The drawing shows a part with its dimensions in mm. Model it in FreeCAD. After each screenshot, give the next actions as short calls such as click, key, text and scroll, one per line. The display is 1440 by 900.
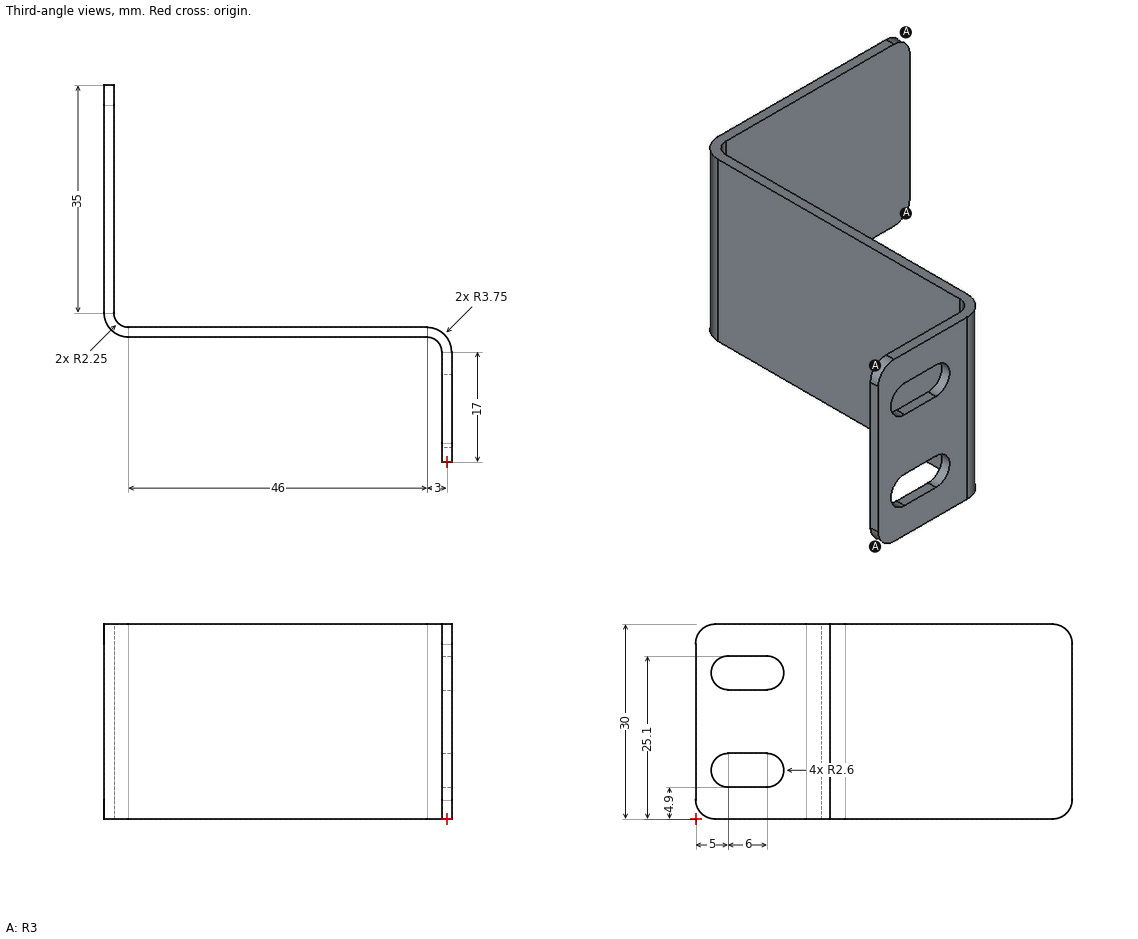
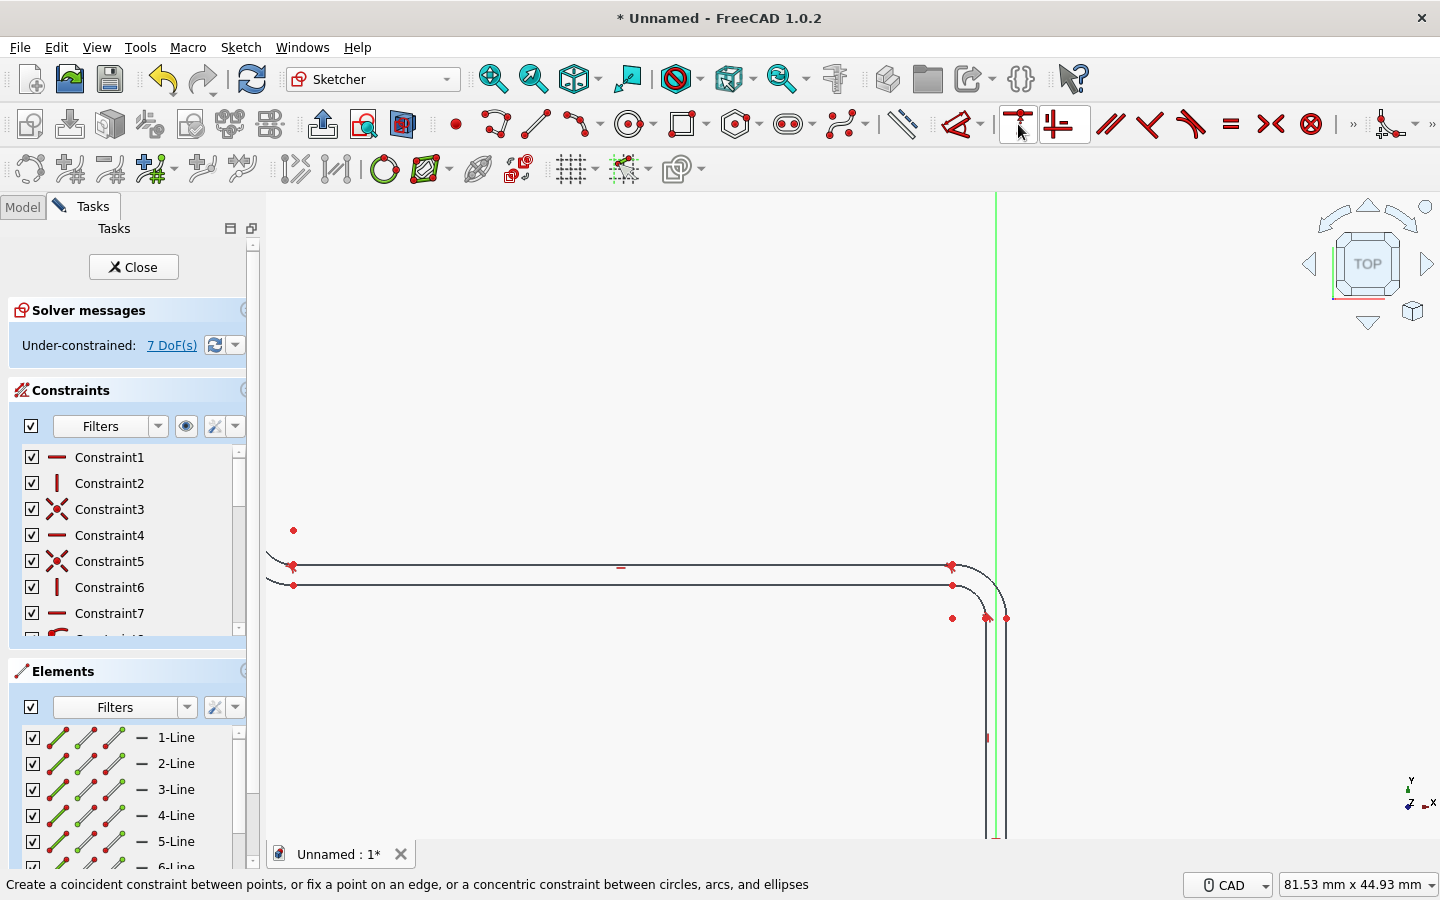
scroll(982, 603, down, 3)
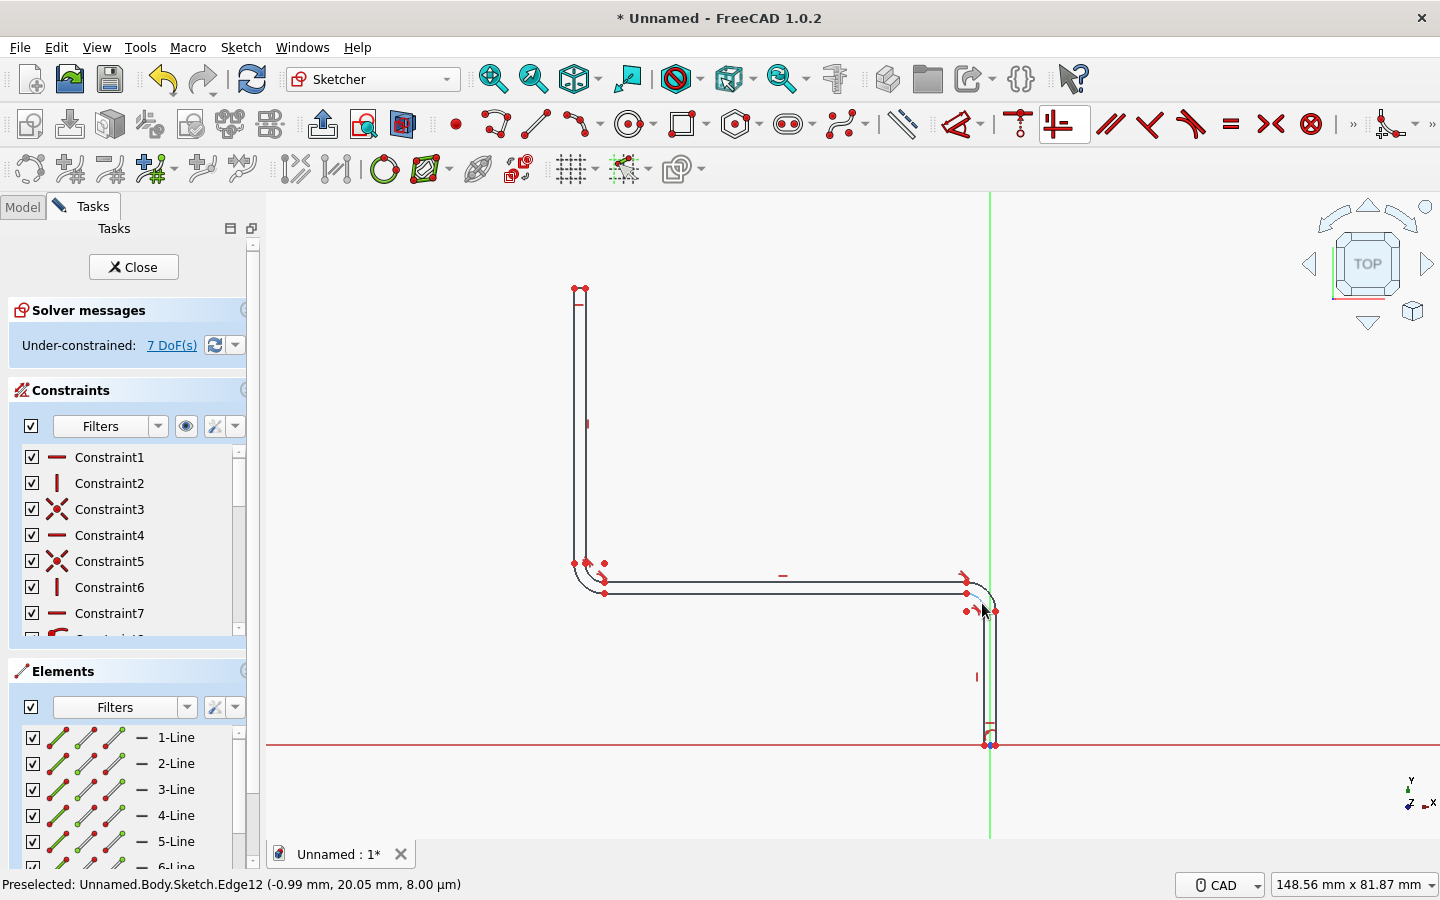
scroll(588, 572, up, 3)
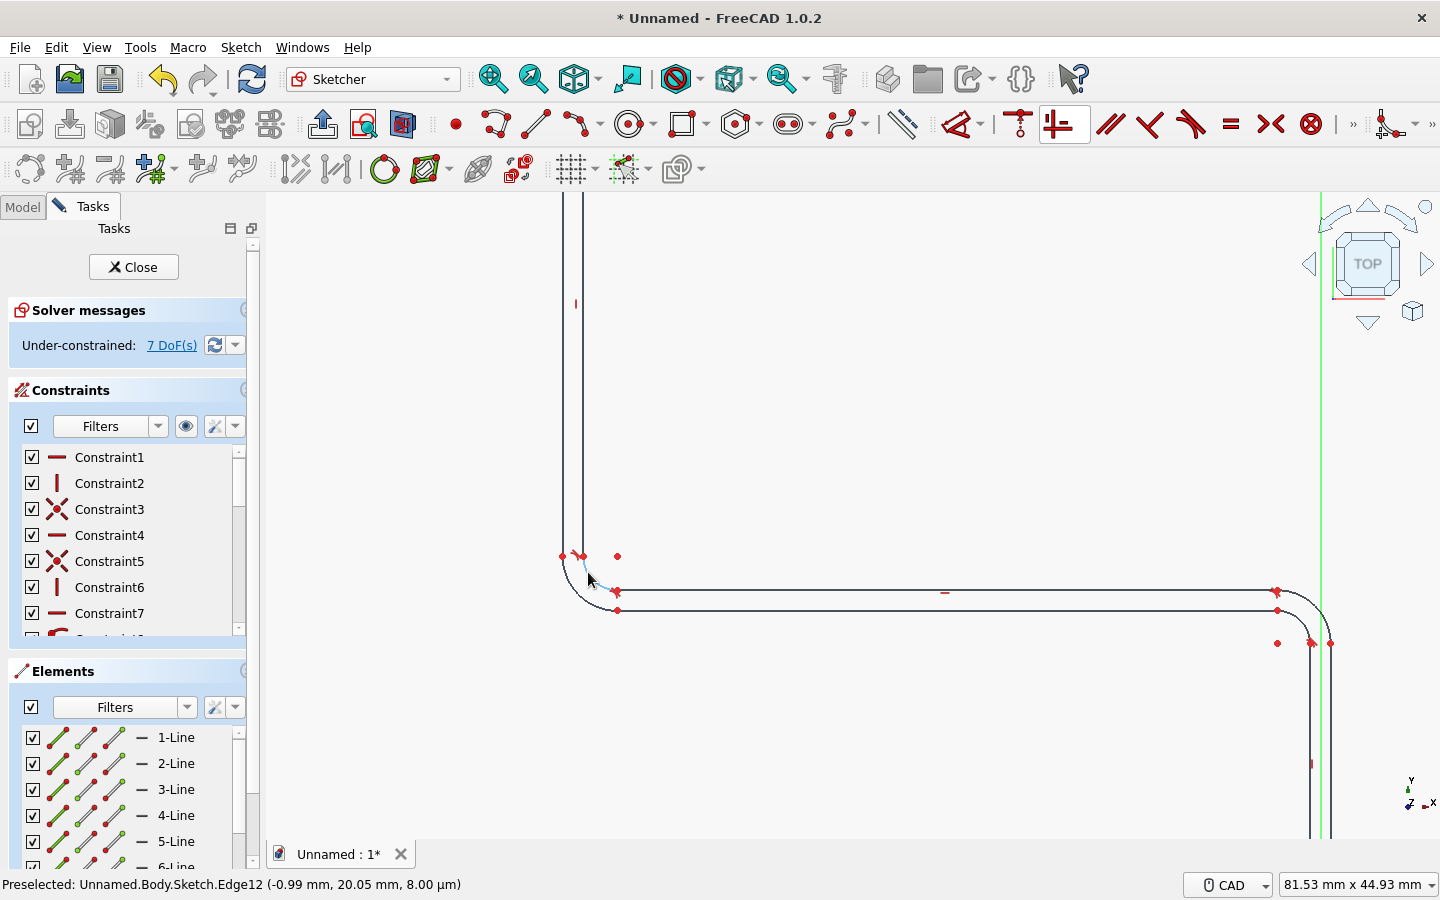
click(587, 572)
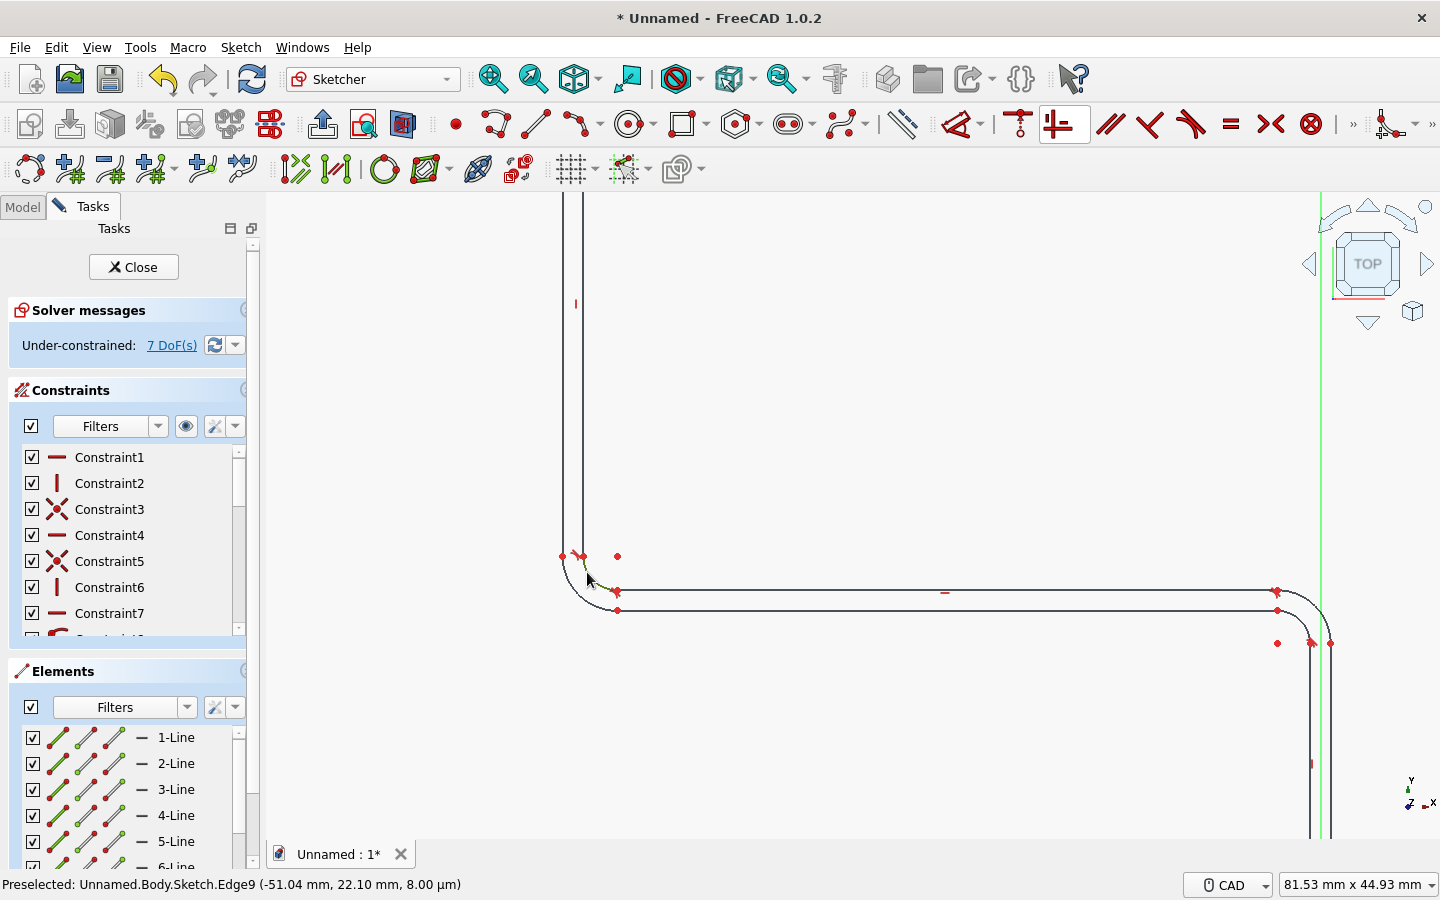
scroll(588, 572, down, 3)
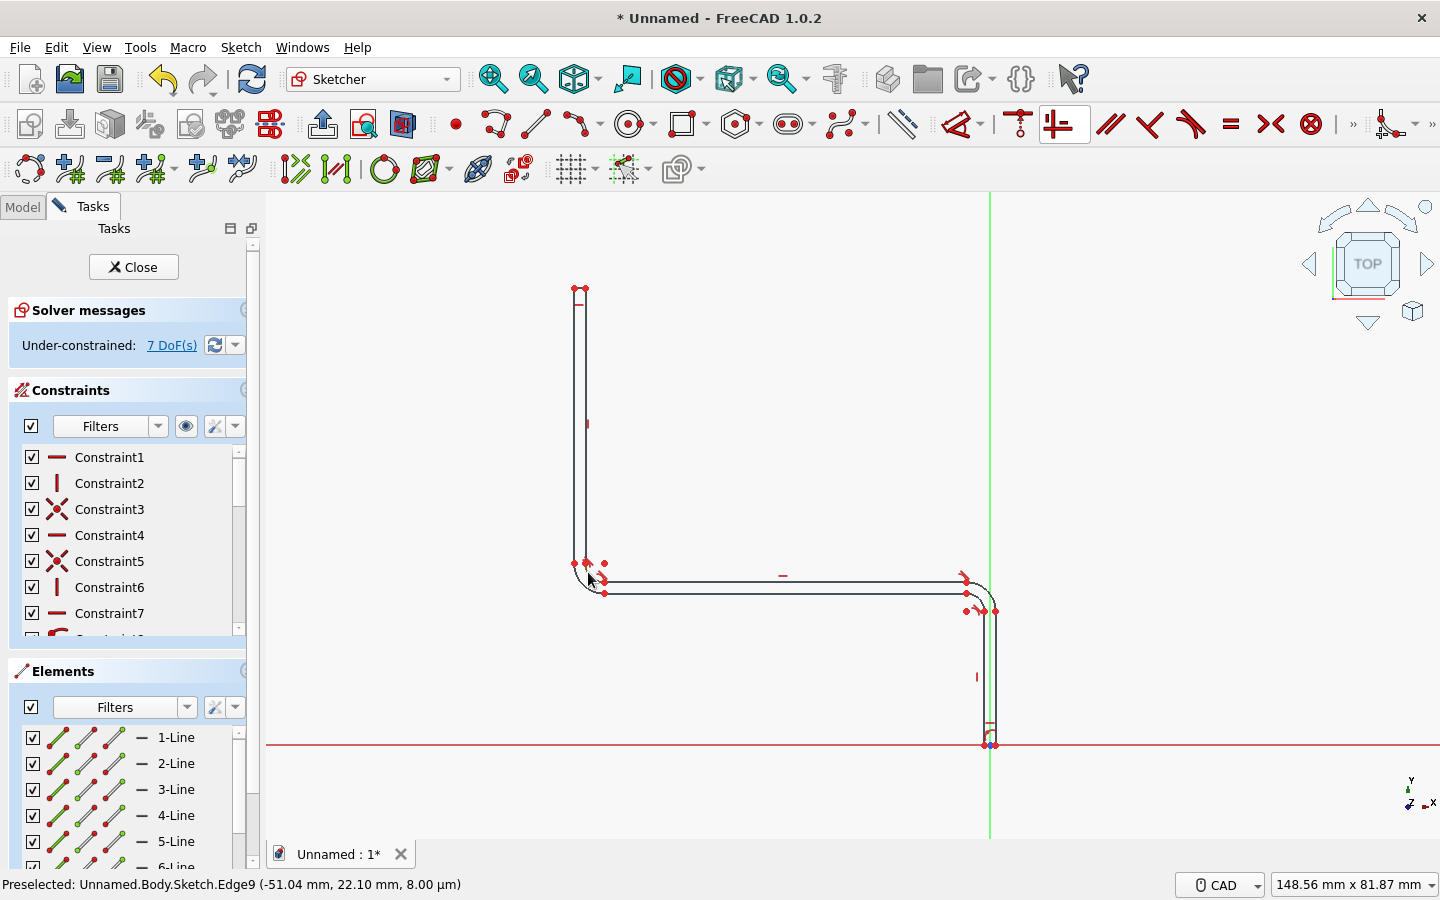
scroll(982, 603, up, 3)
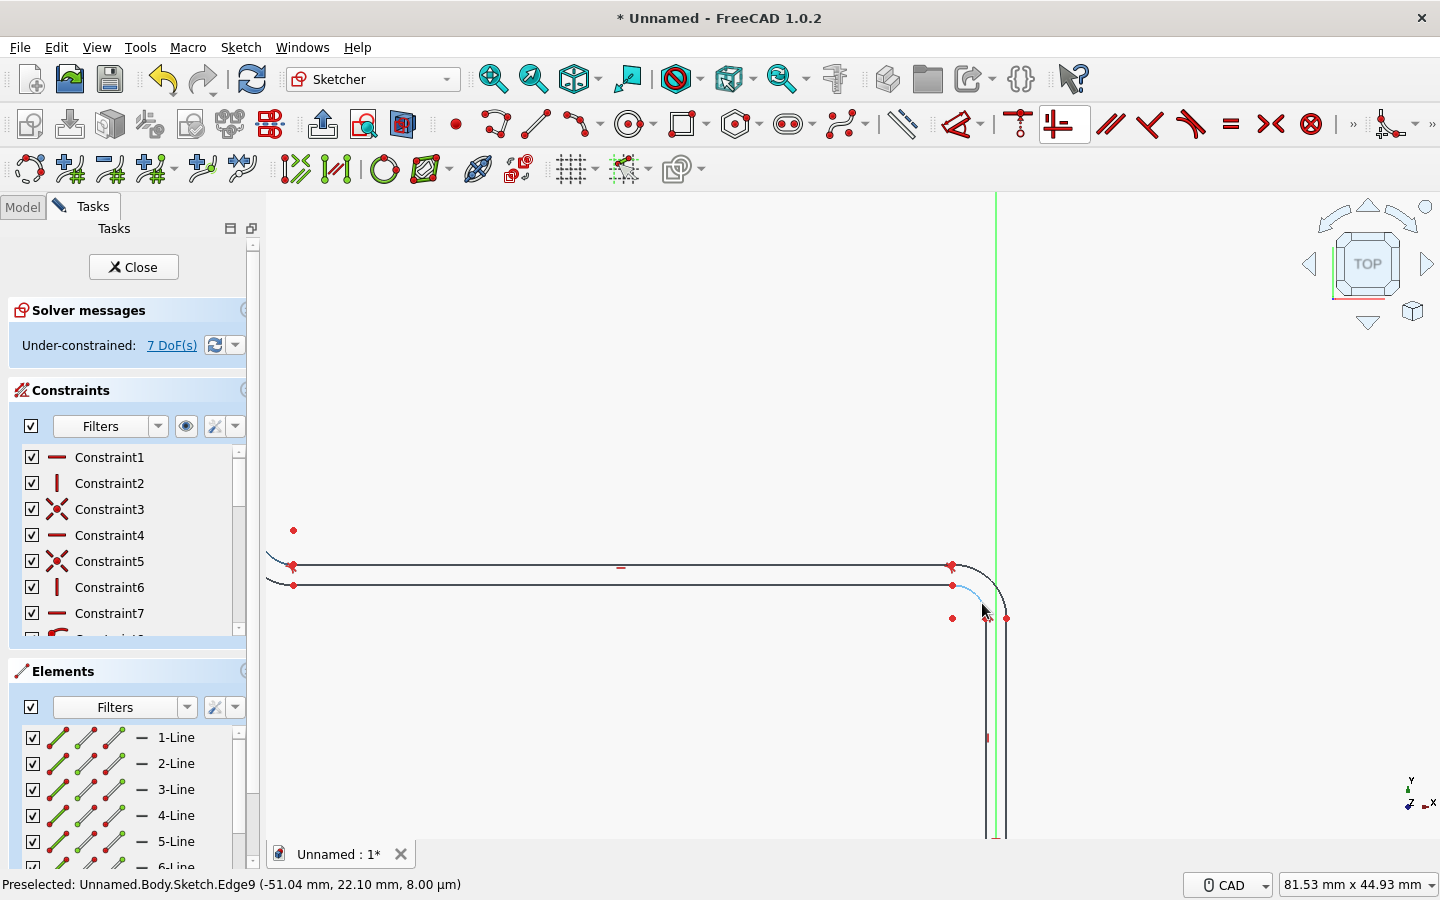
click(982, 603)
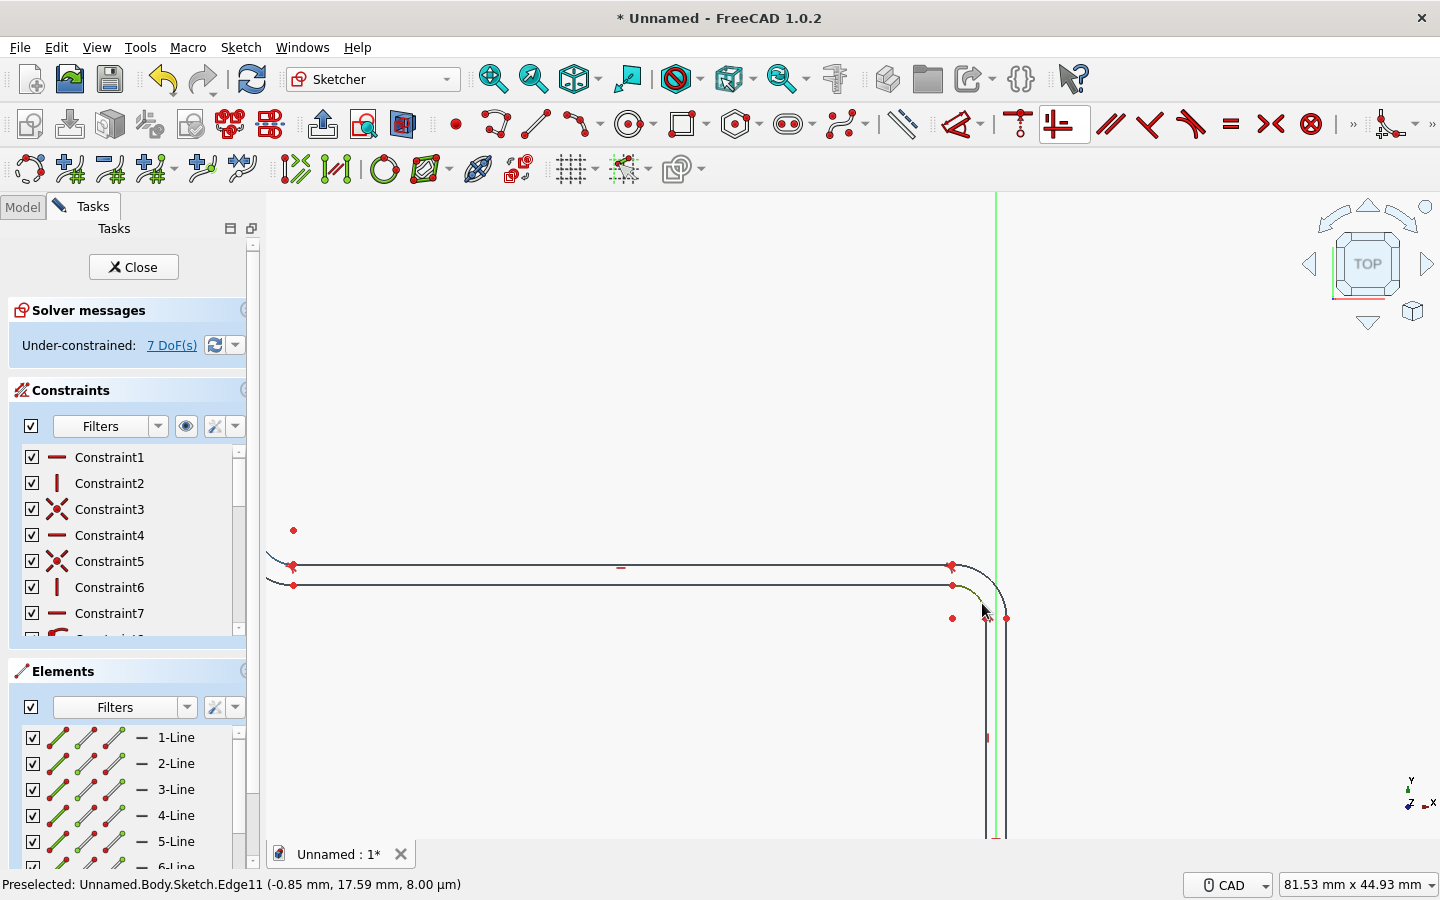
key(e)